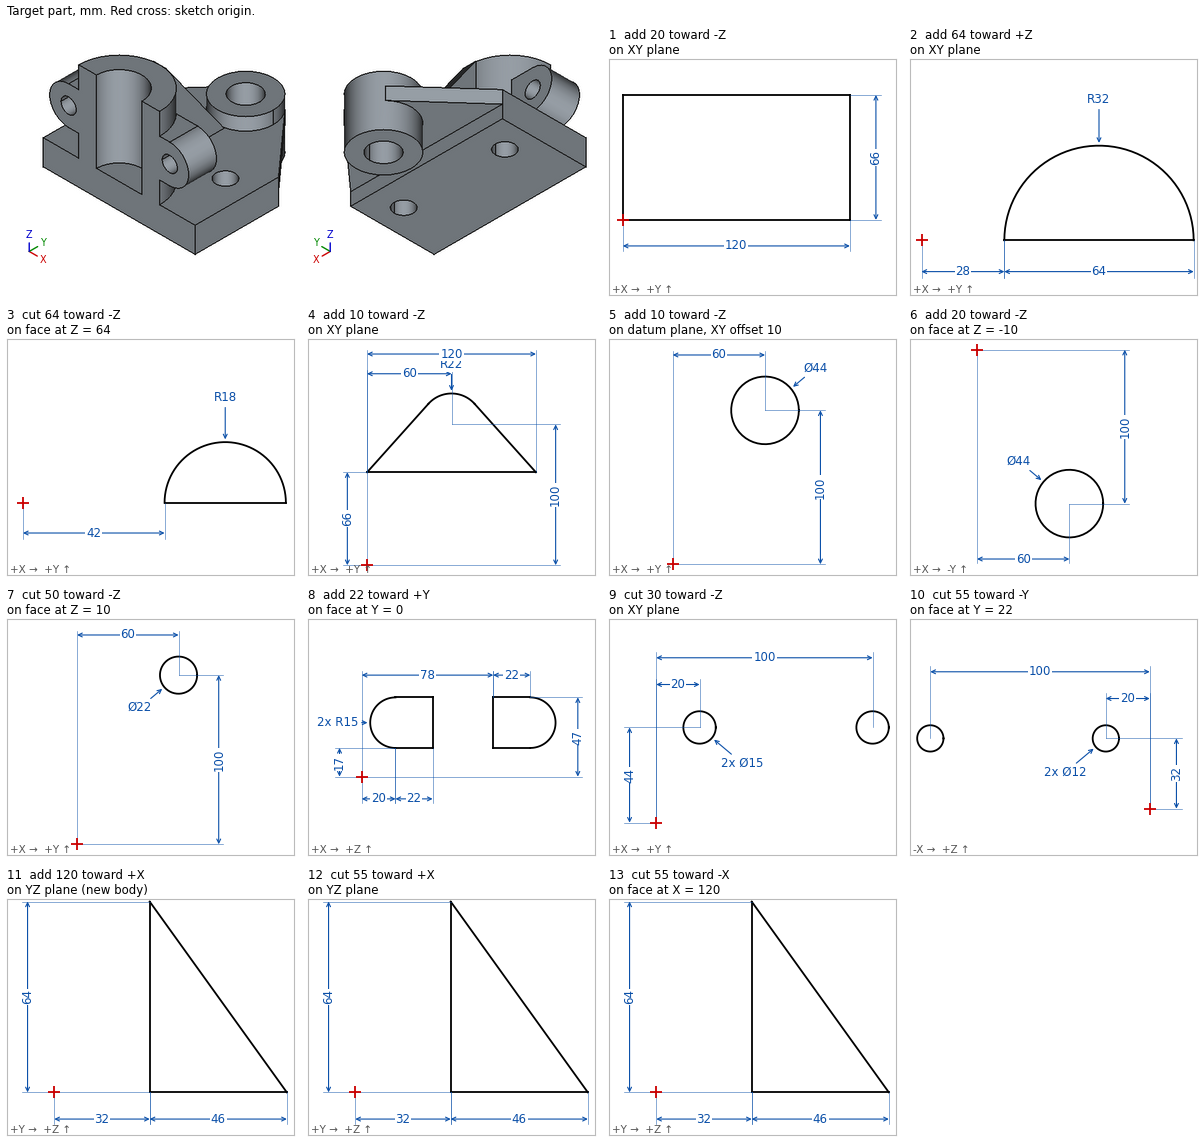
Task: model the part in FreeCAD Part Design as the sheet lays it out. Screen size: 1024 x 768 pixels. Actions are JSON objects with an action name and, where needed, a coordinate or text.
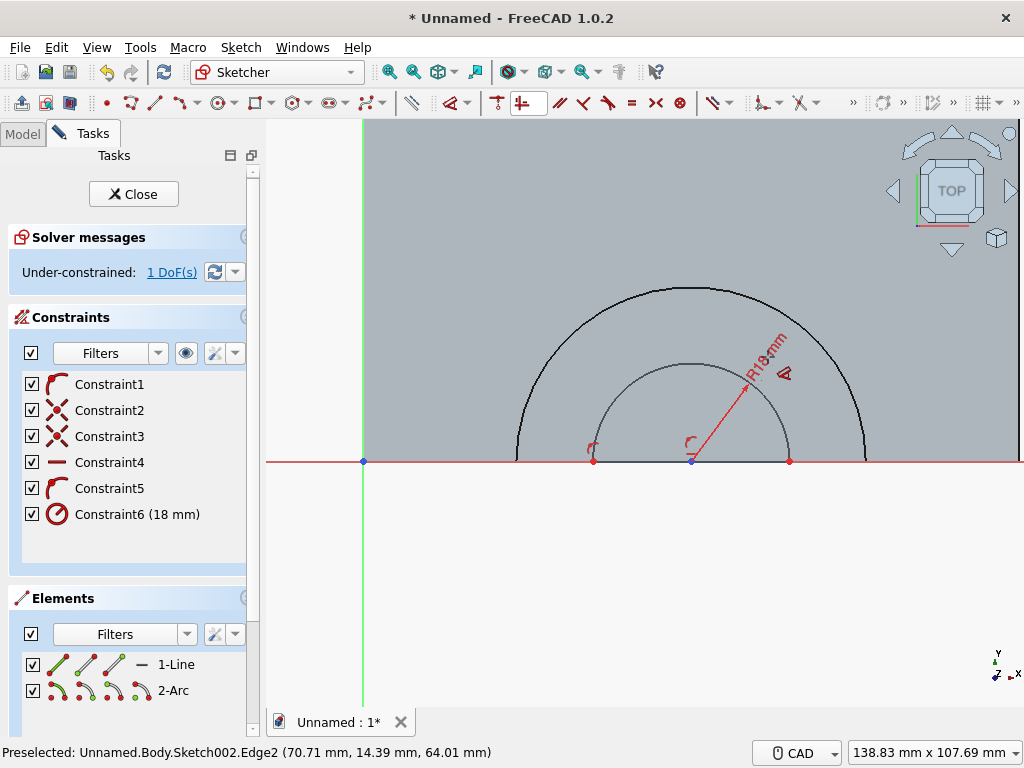
{"action": "left_click", "coordinate": [593, 462]}
{"action": "left_click", "coordinate": [478, 496]}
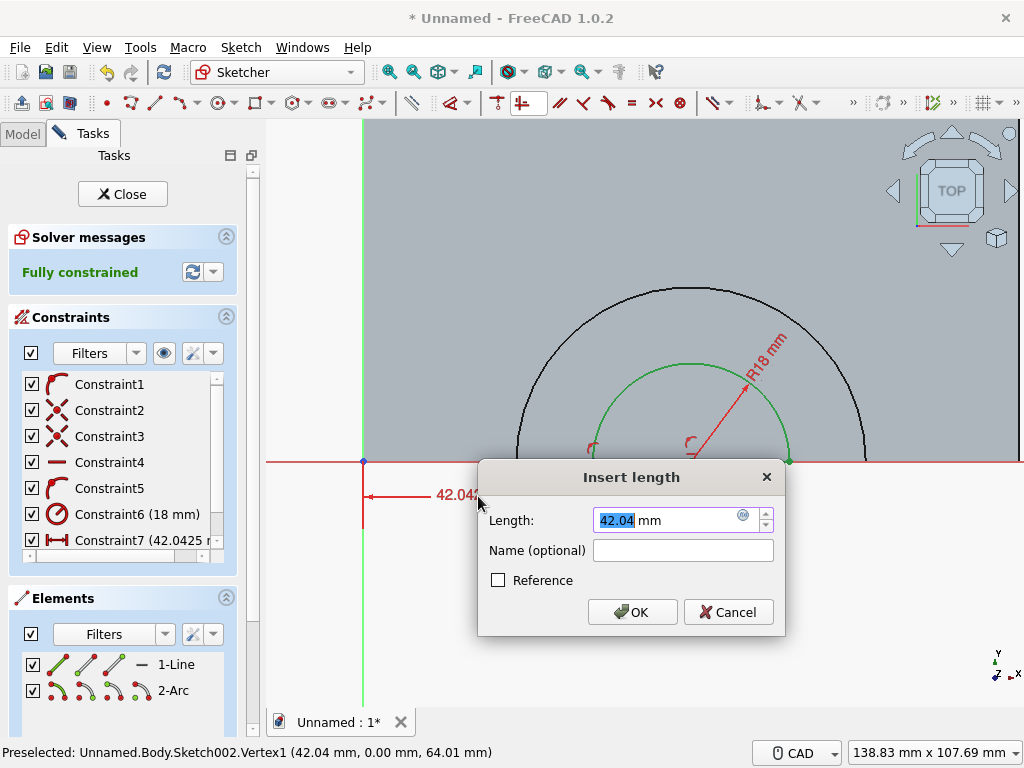
{"action": "type", "text": "42"}
{"action": "key", "text": "Return"}
{"action": "key", "text": "Escape"}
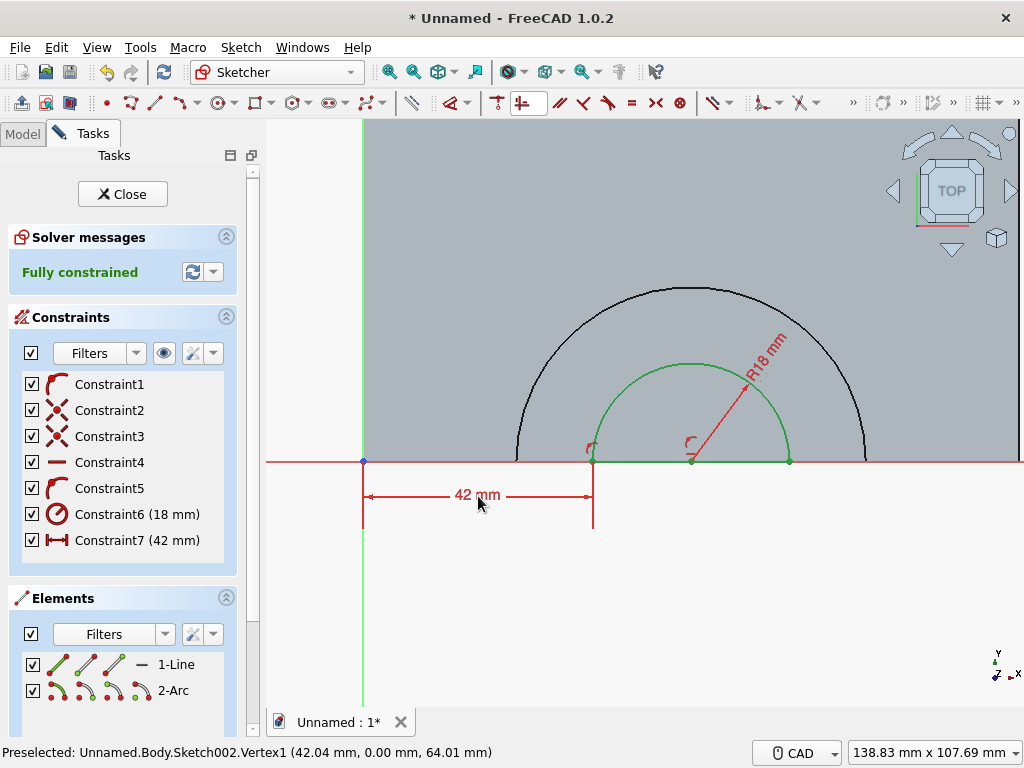
{"action": "left_click", "coordinate": [123, 194]}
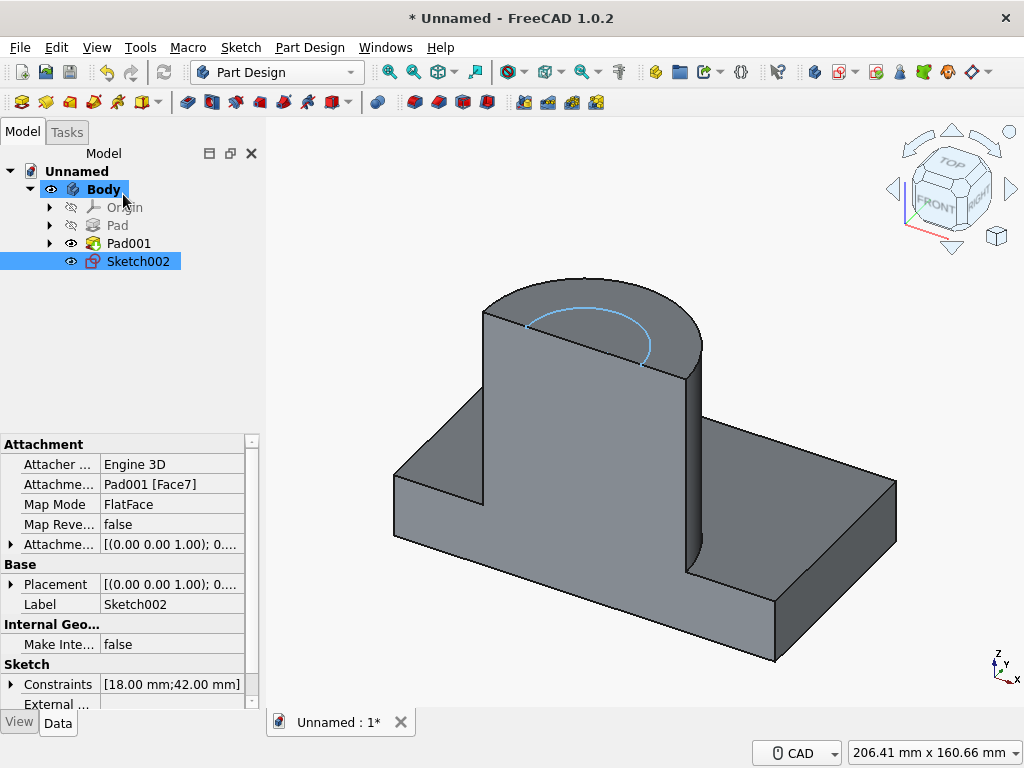
{"action": "left_click", "coordinate": [188, 102]}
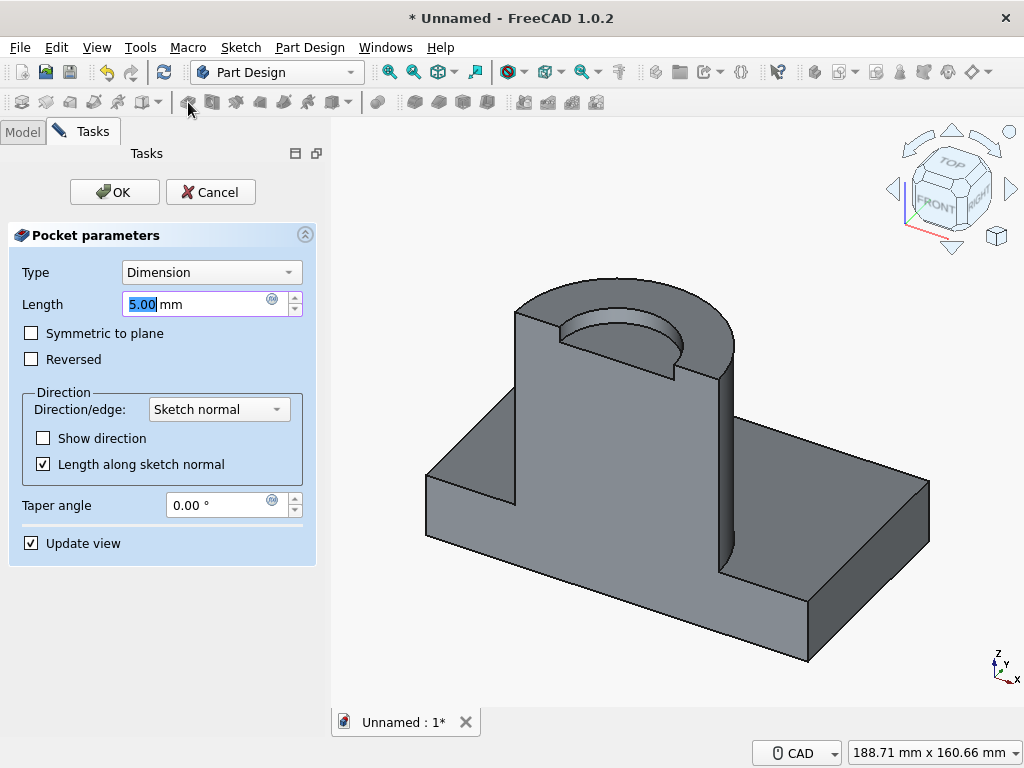
{"action": "type", "text": "64"}
{"action": "key", "text": "Tab"}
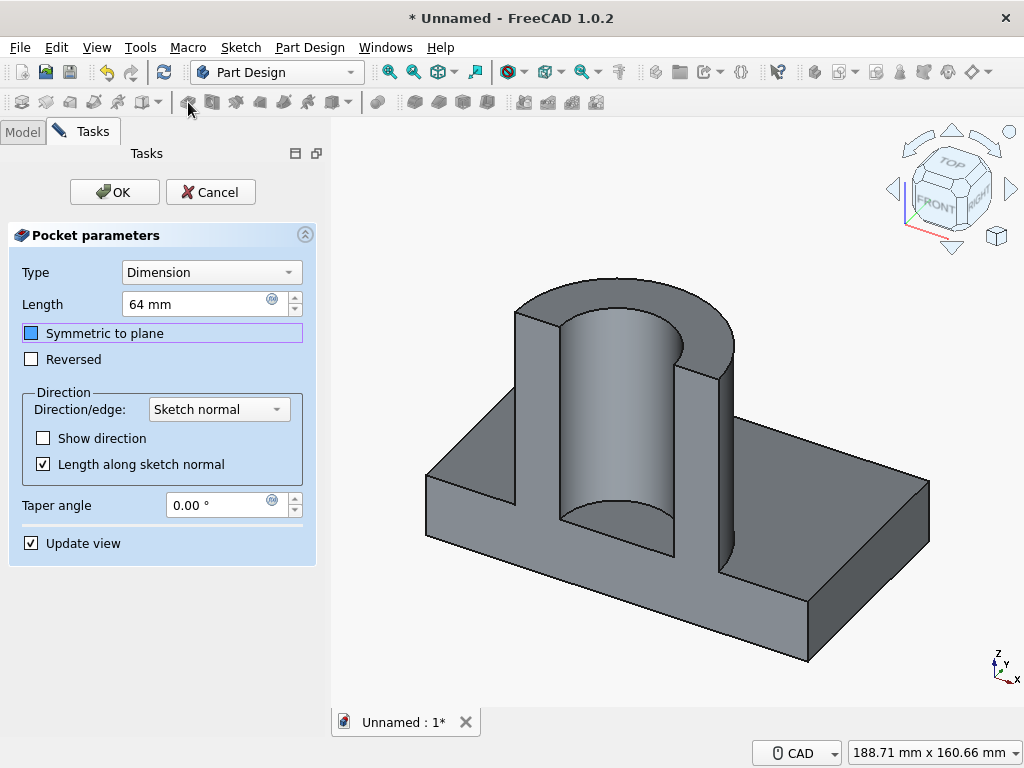
{"action": "left_click", "coordinate": [115, 192]}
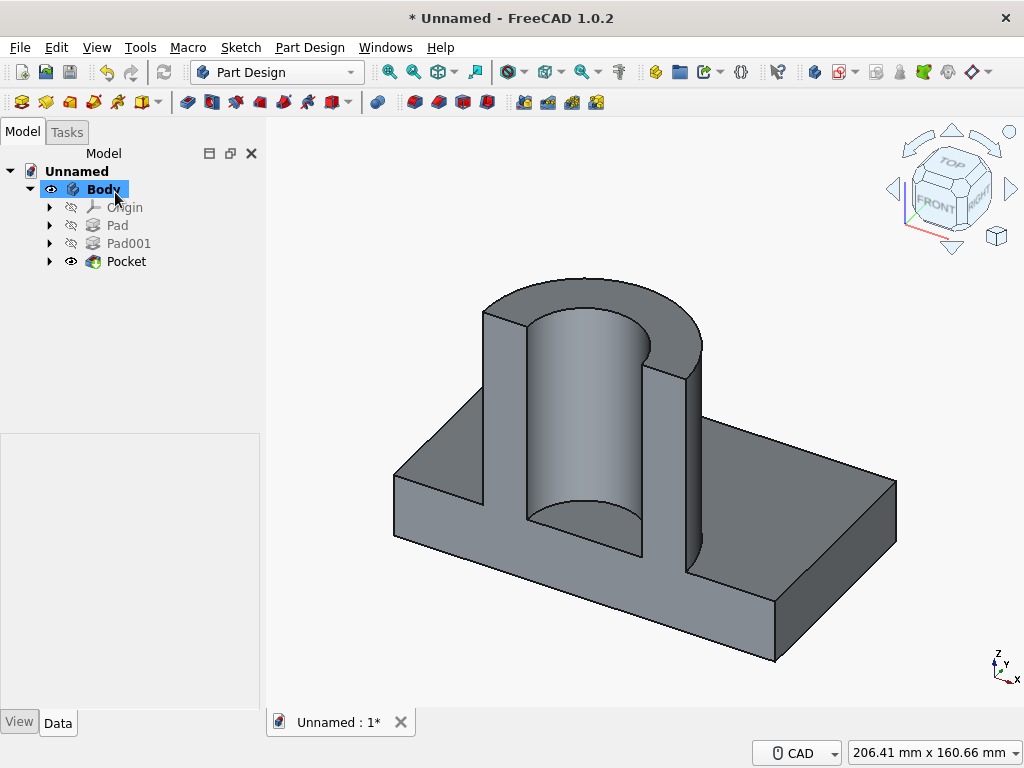
{"action": "left_click", "coordinate": [840, 72]}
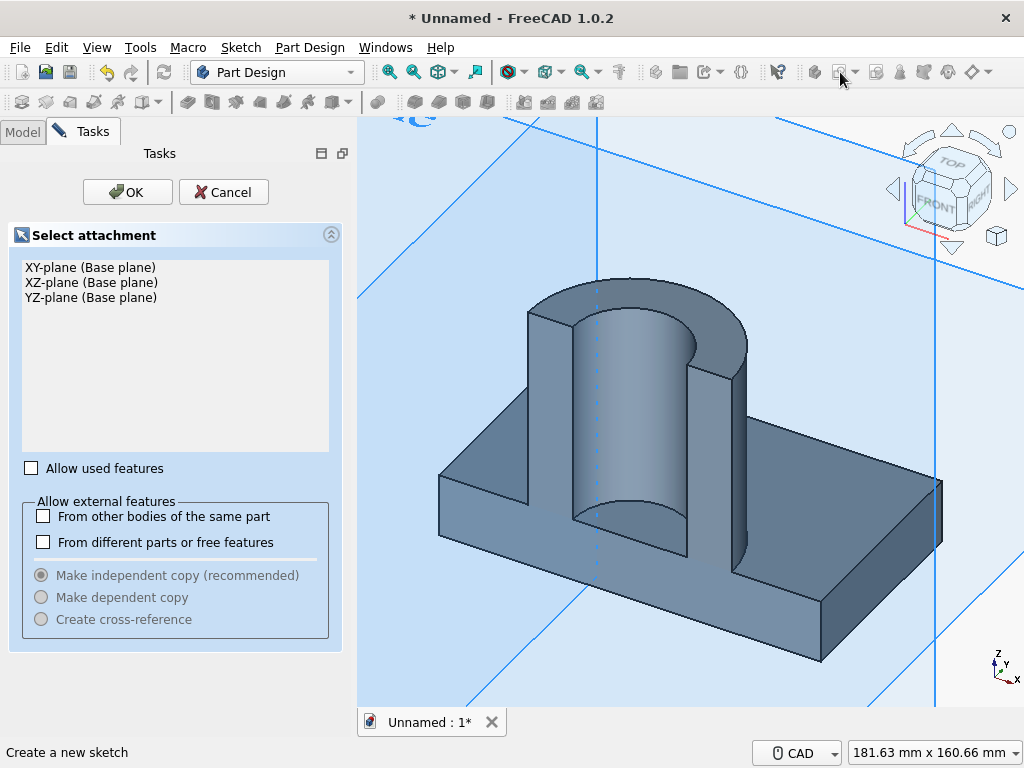
{"action": "left_click", "coordinate": [82, 268]}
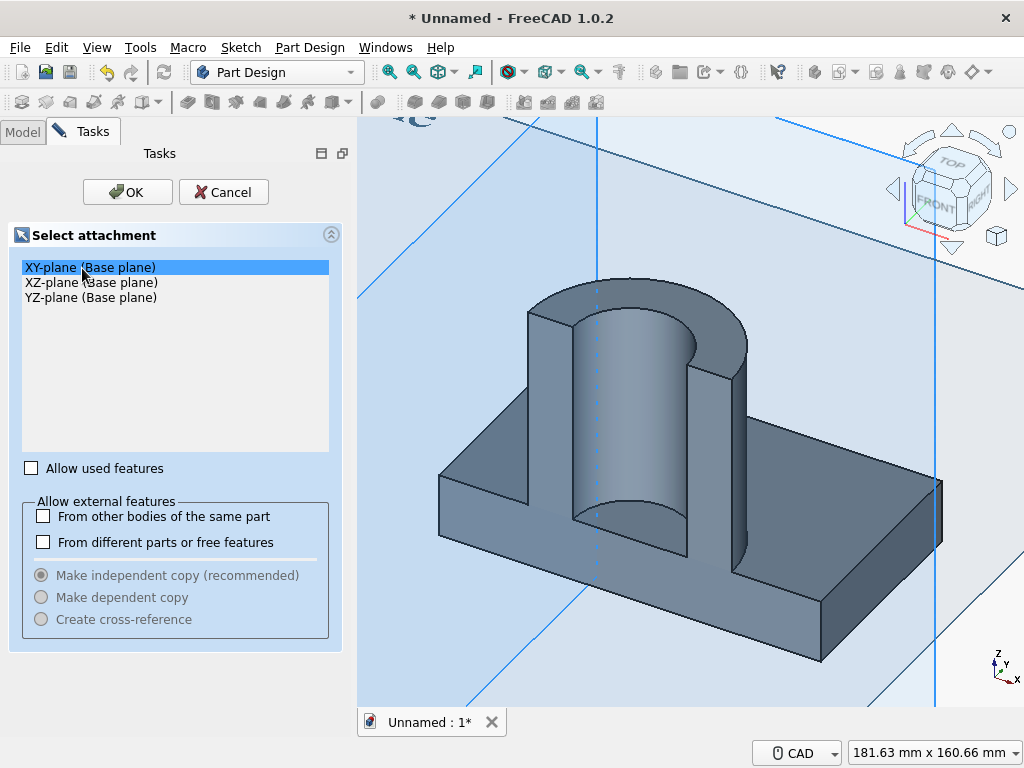
{"action": "left_click", "coordinate": [128, 192]}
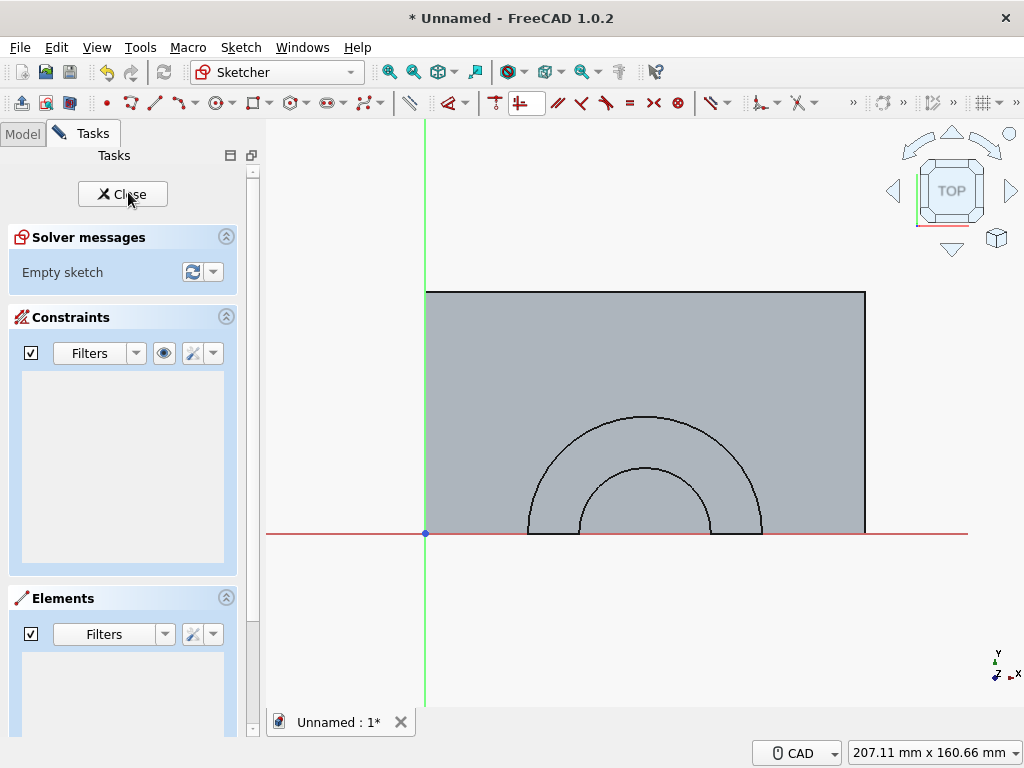
{"action": "left_click", "coordinate": [70, 104]}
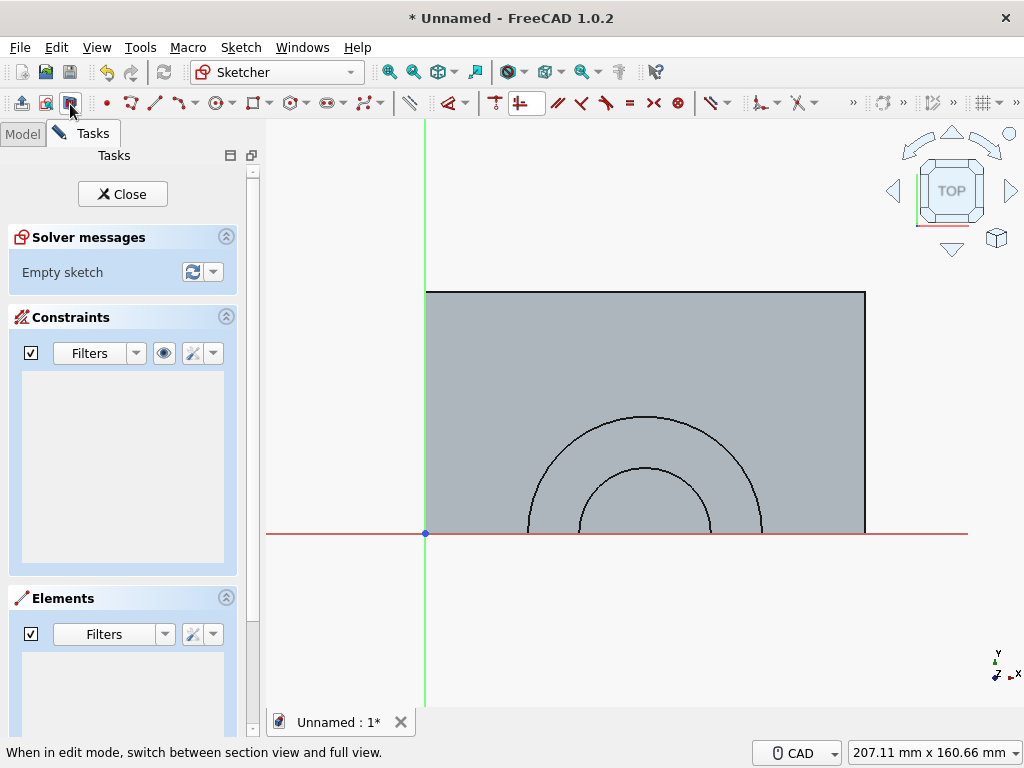
{"action": "scroll", "coordinate": [294, 679], "scroll_direction": "down", "scroll_amount": 1}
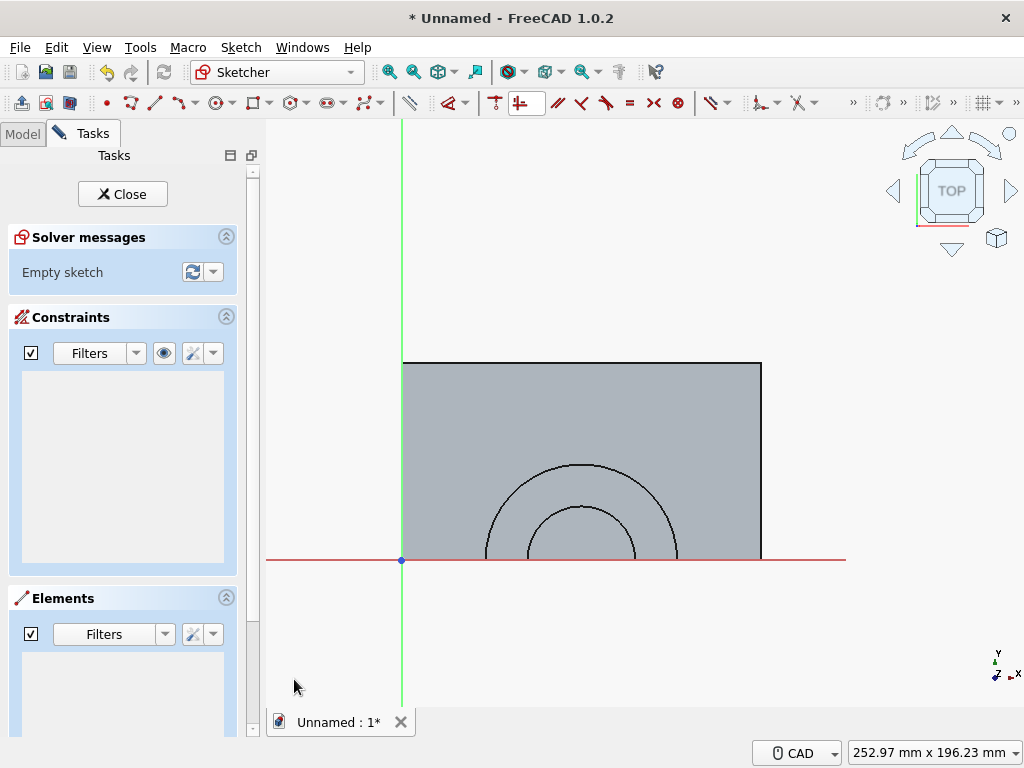
{"action": "left_click", "coordinate": [132, 104]}